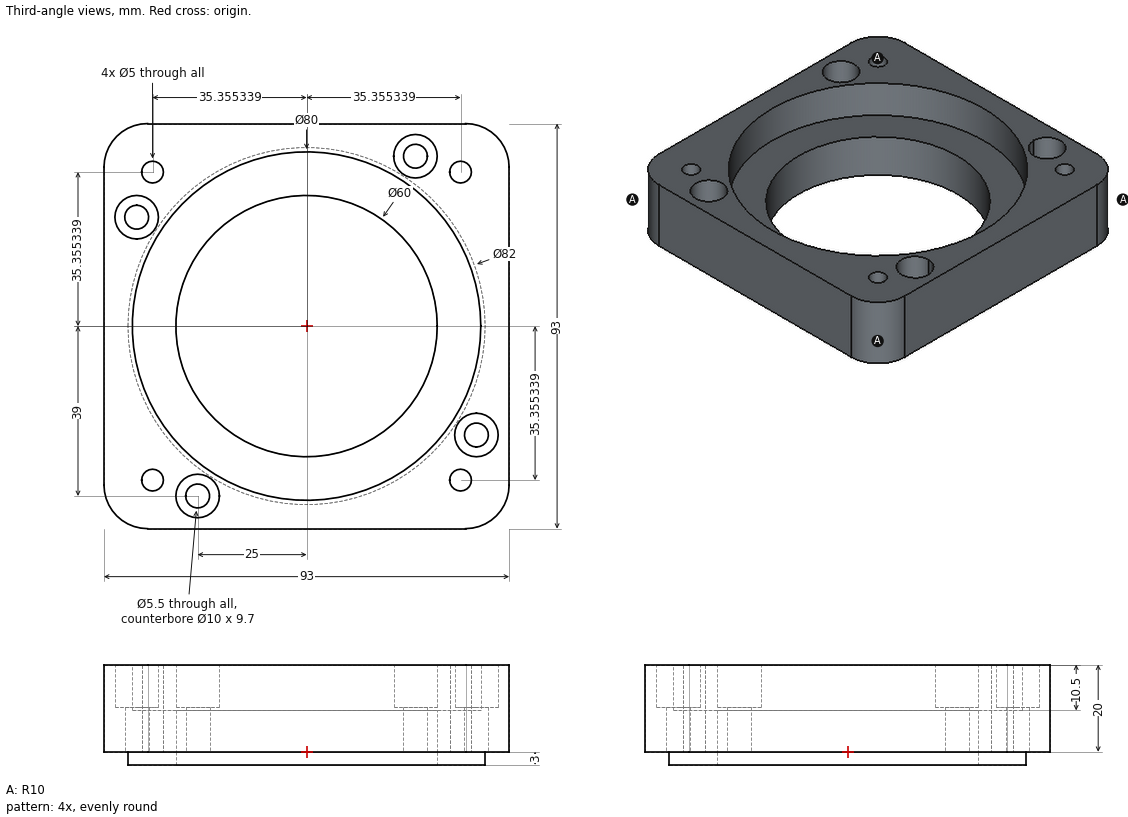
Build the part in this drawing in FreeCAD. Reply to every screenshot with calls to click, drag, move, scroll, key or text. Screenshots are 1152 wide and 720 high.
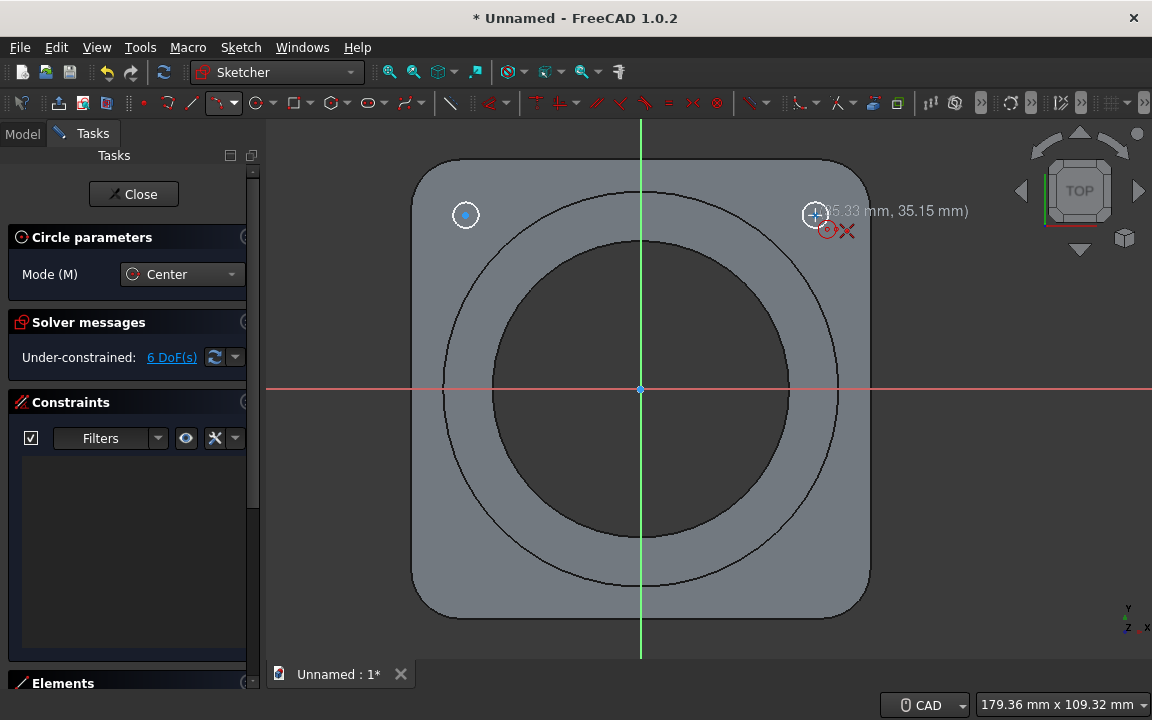
scroll(815, 564, up, 4)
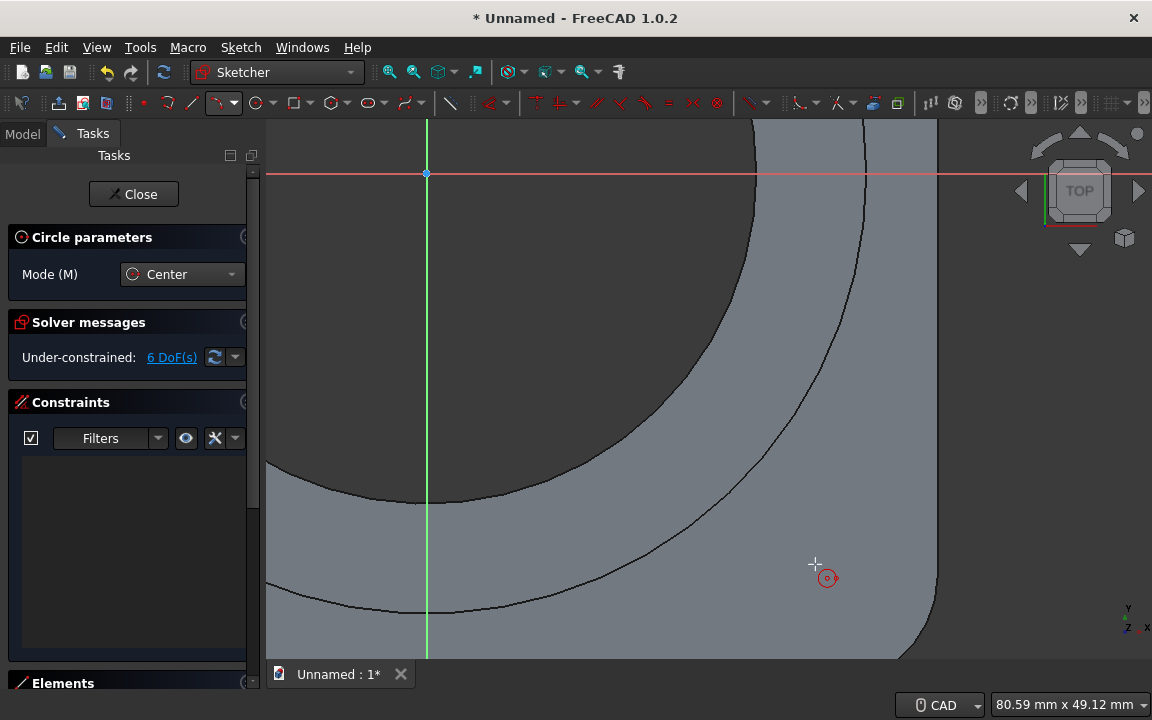
click(815, 563)
click(835, 543)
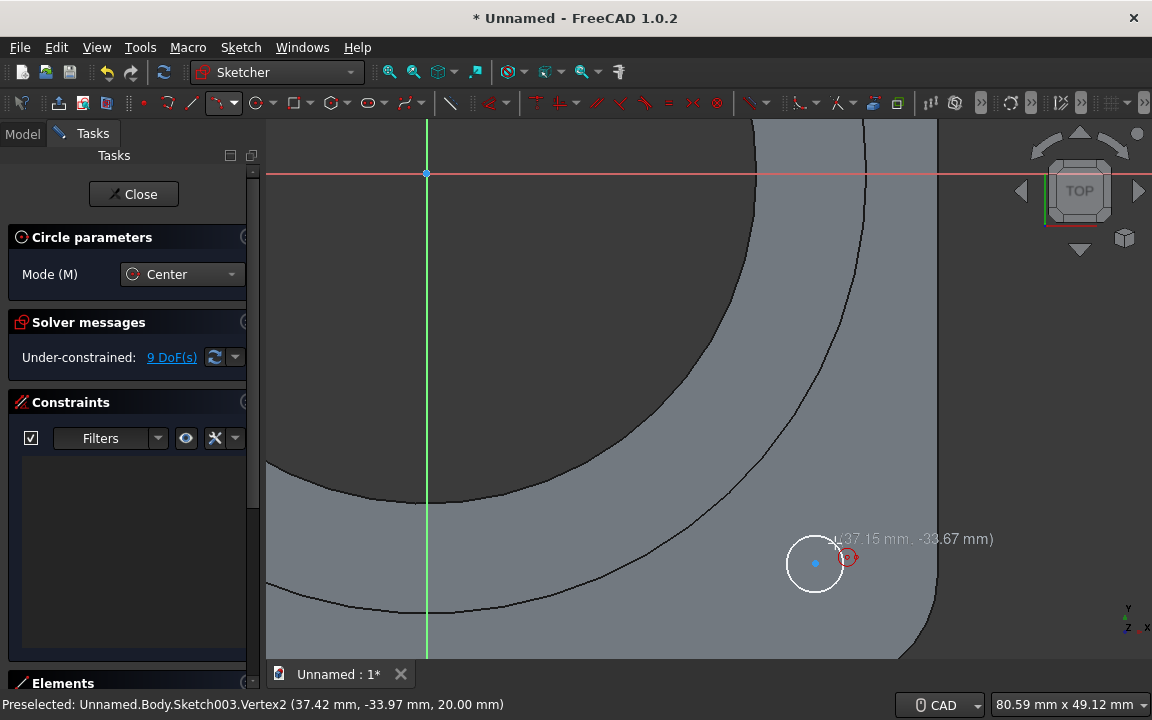
scroll(815, 565, down, 4)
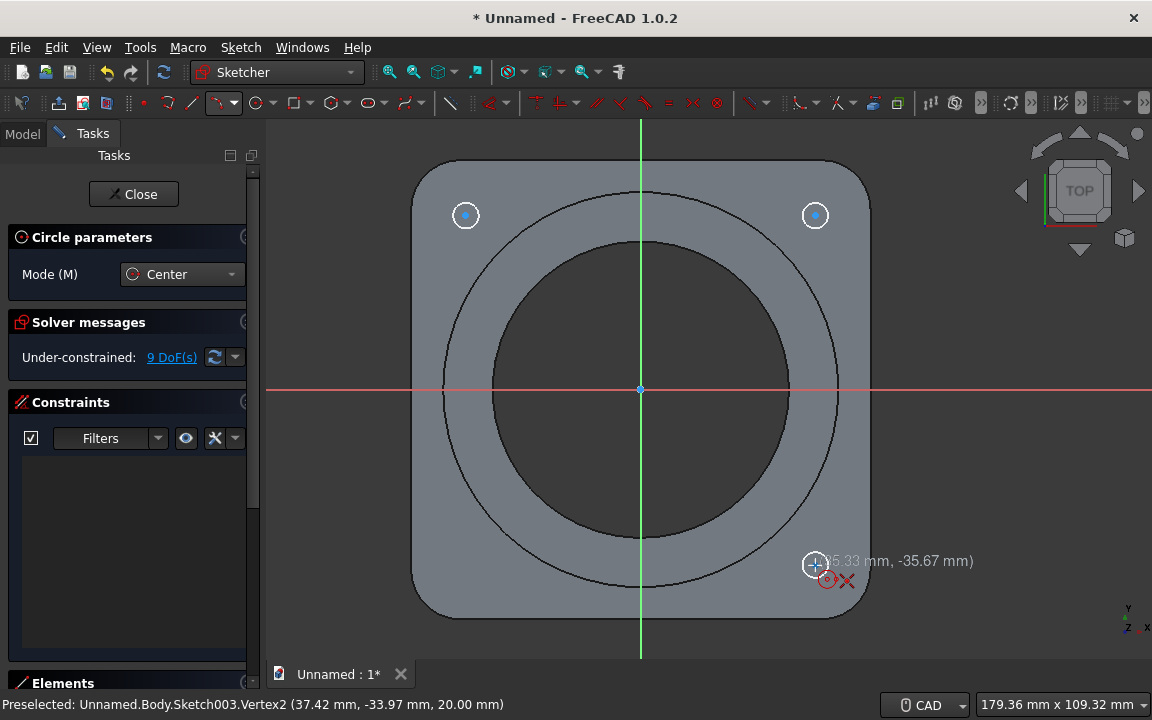
scroll(466, 564, up, 4)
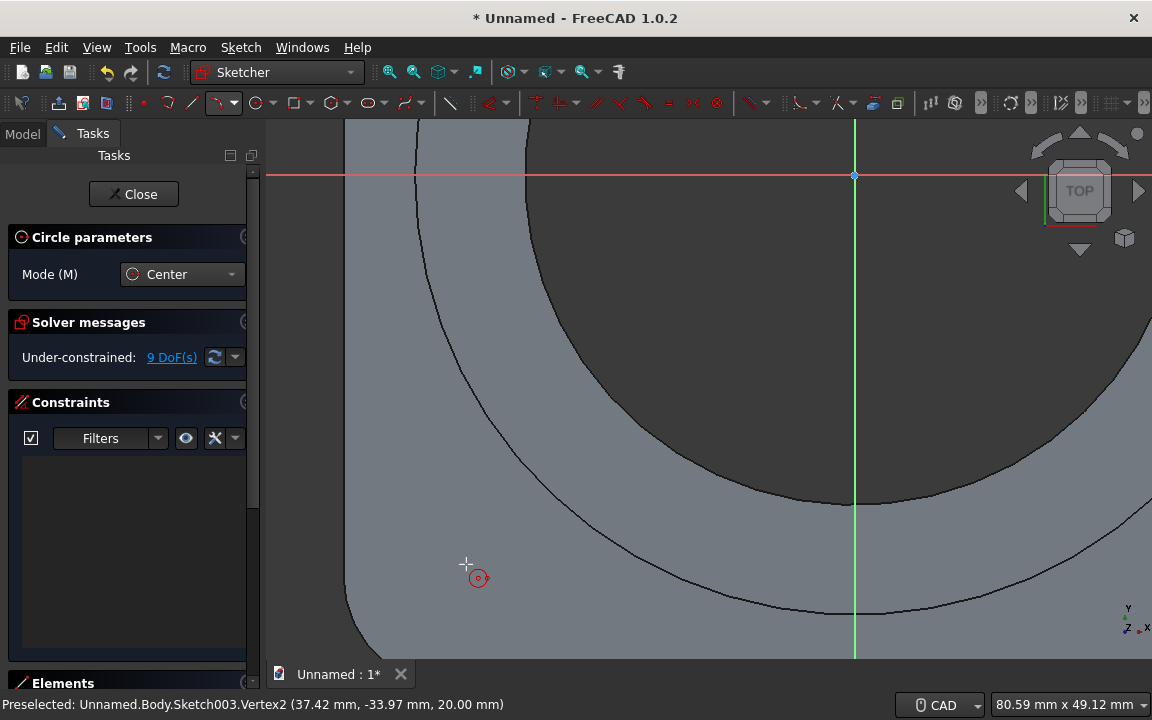
click(466, 564)
click(485, 544)
key(Escape)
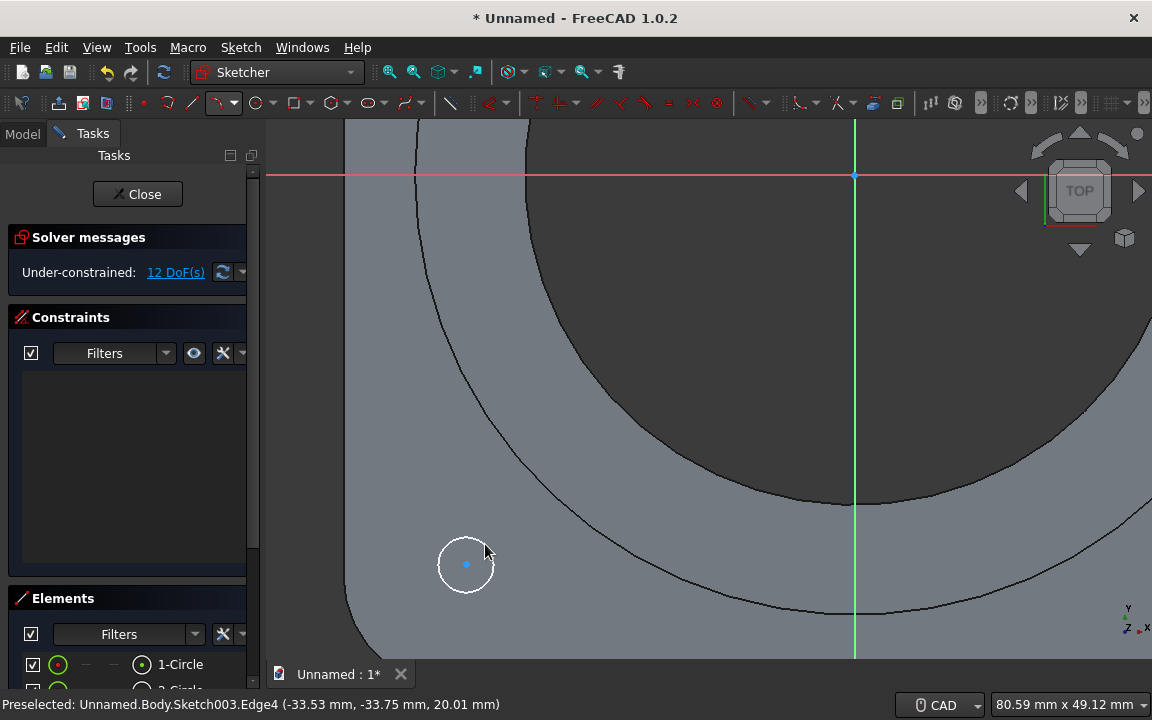
scroll(466, 564, down, 4)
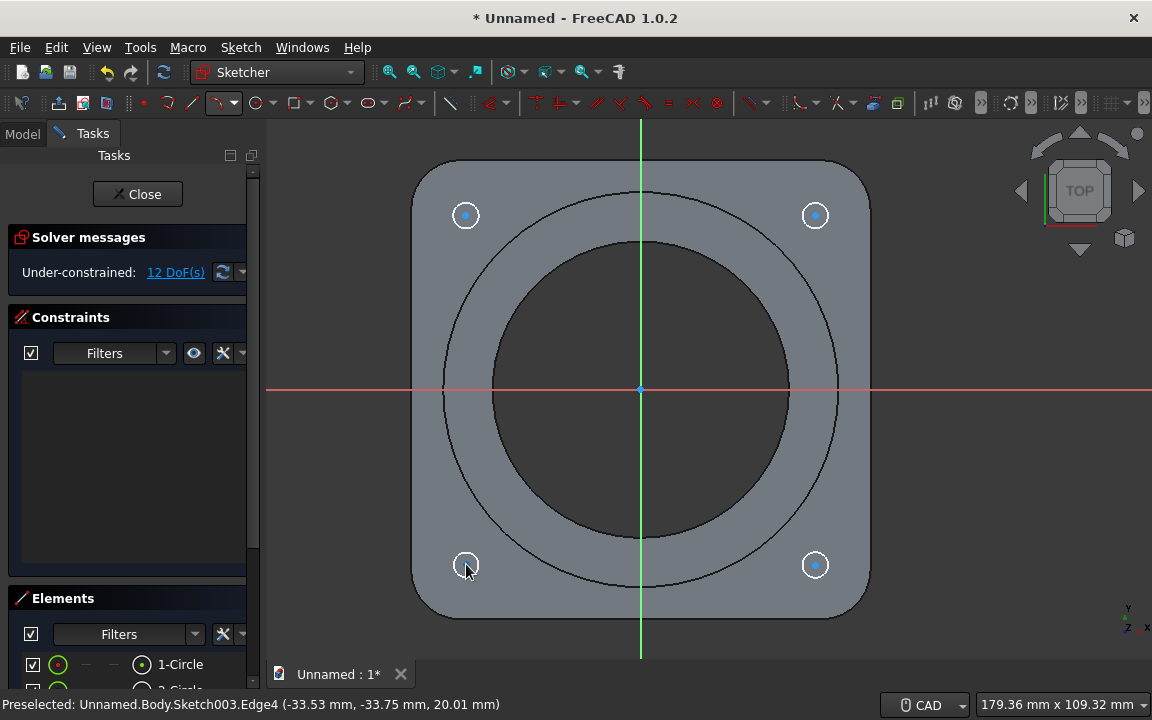
click(475, 207)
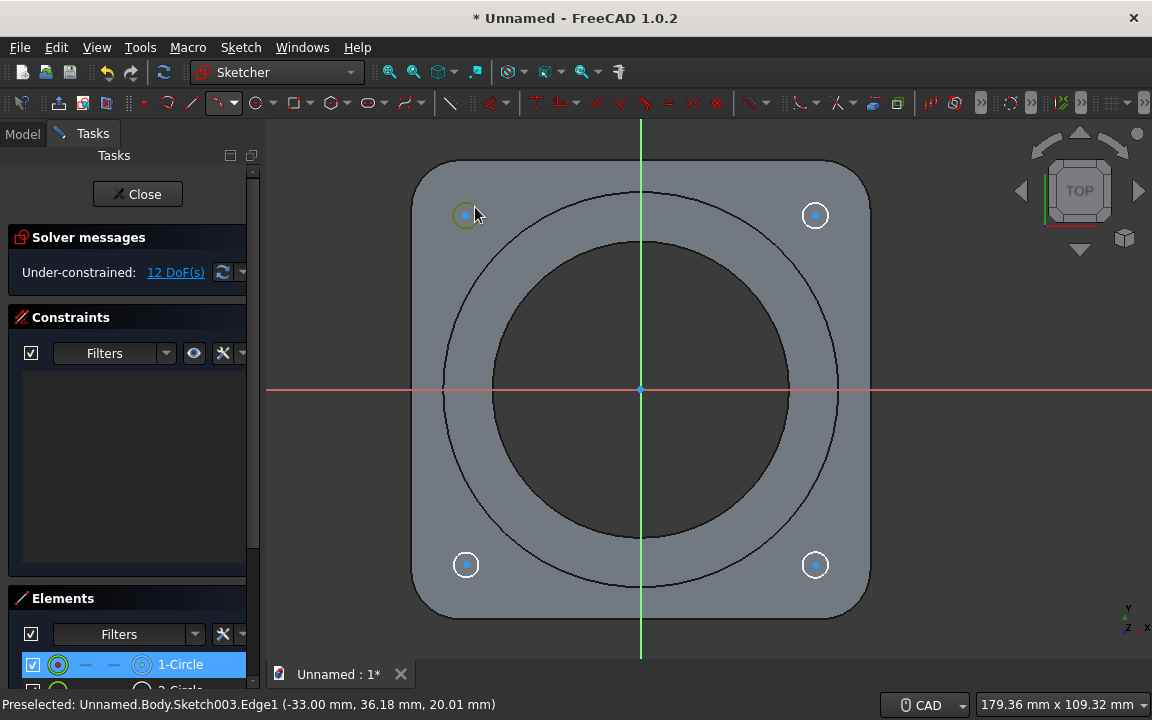
click(824, 207)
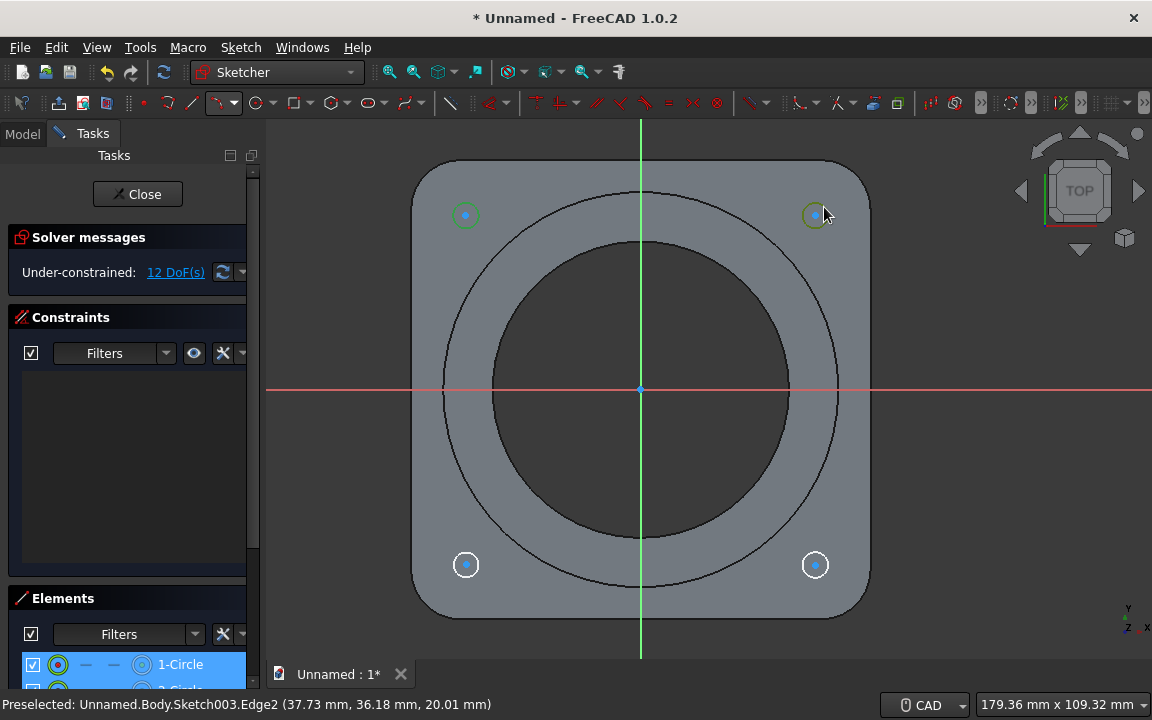
click(824, 556)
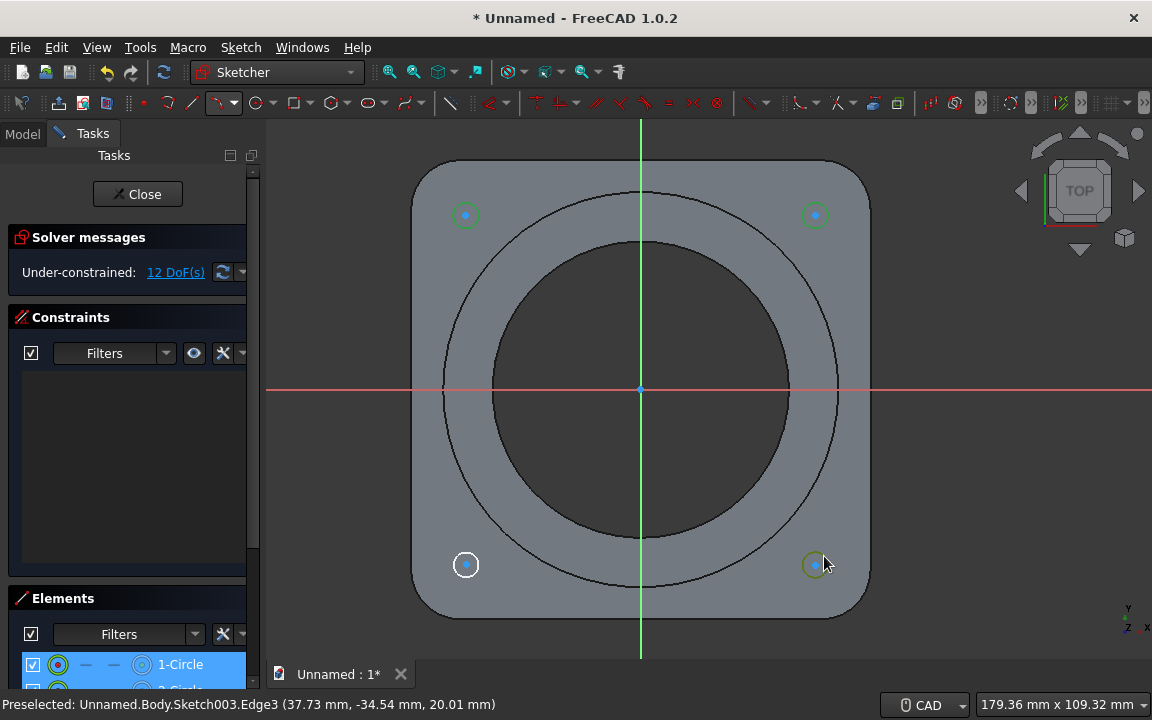
click(475, 556)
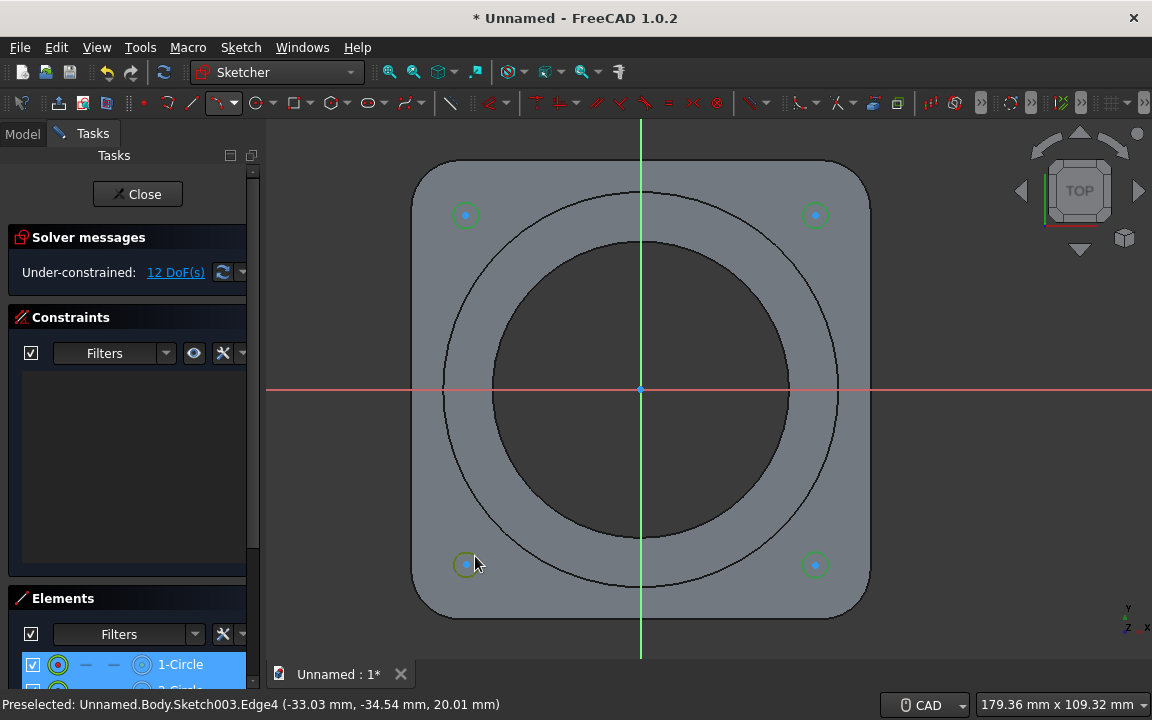
click(670, 104)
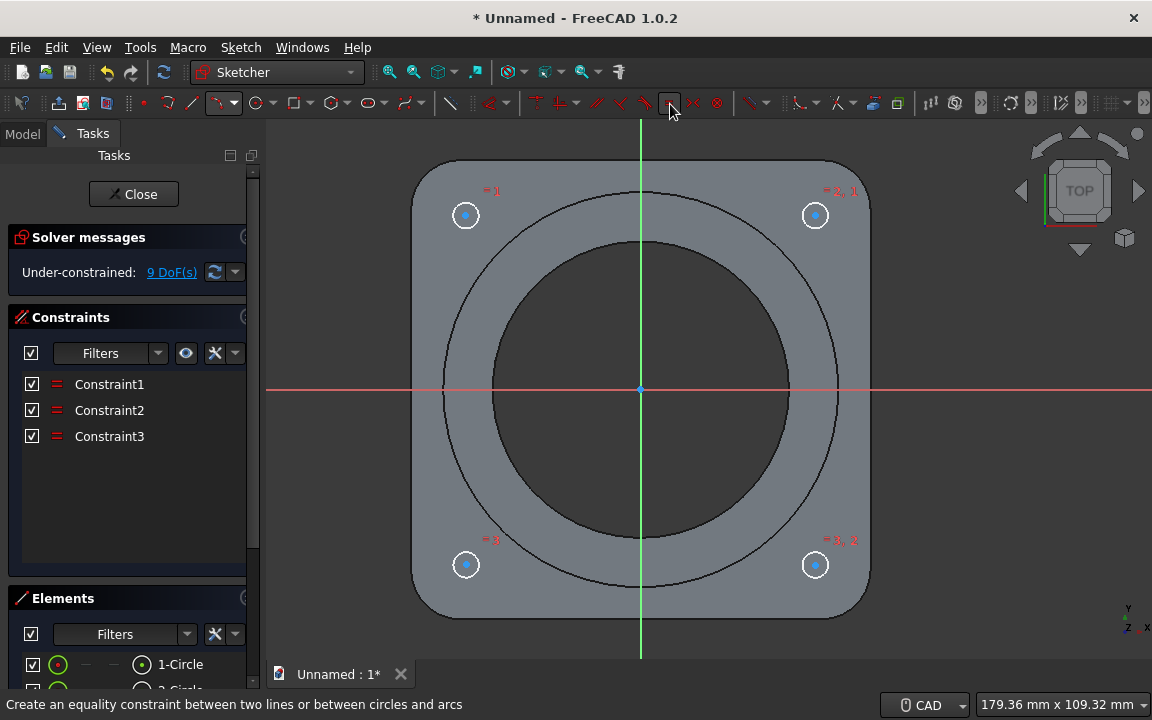
click(466, 216)